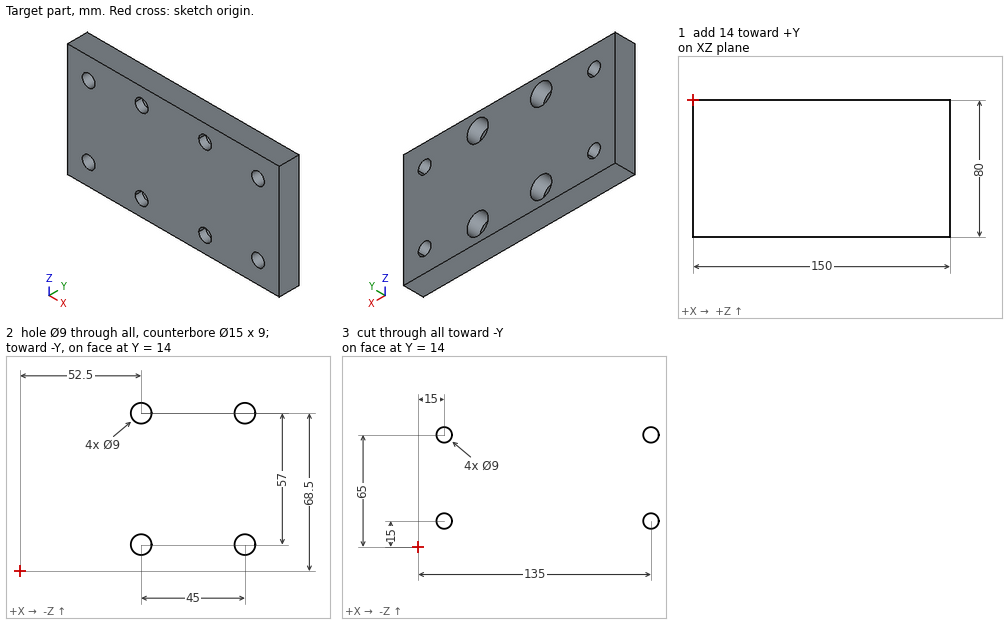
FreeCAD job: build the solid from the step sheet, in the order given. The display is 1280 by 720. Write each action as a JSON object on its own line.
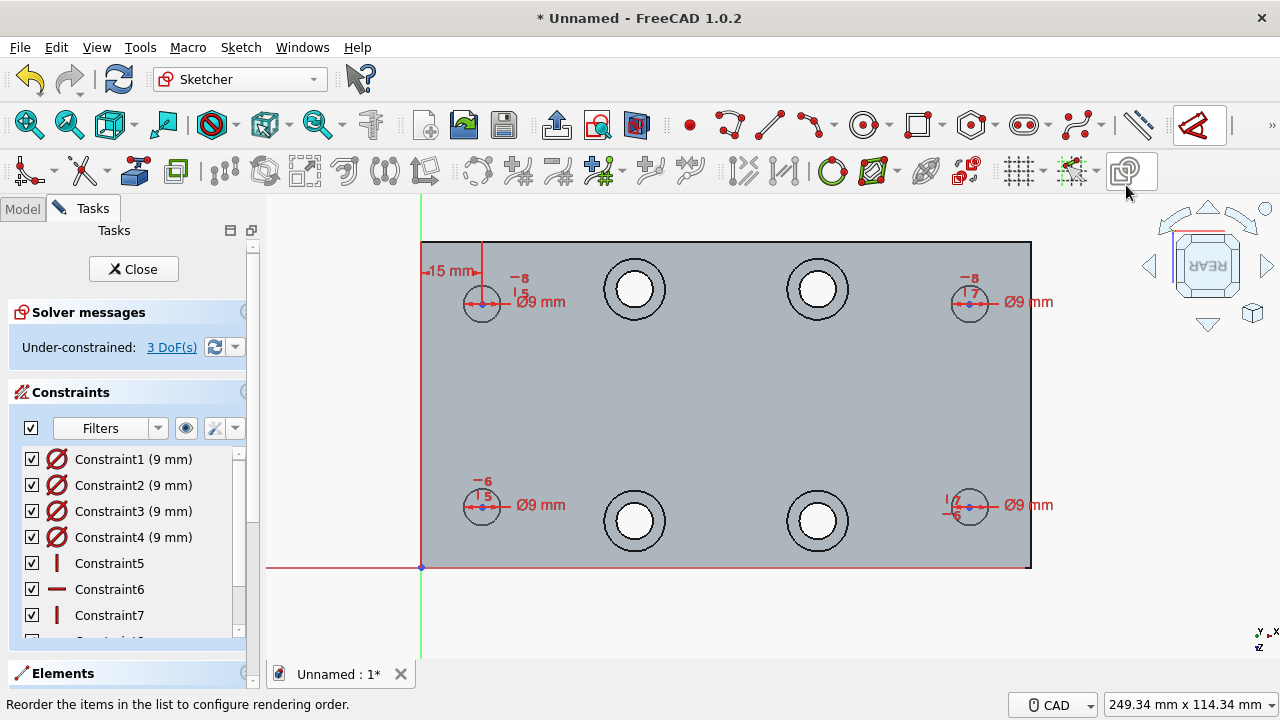
{"action": "left_click", "coordinate": [482, 304]}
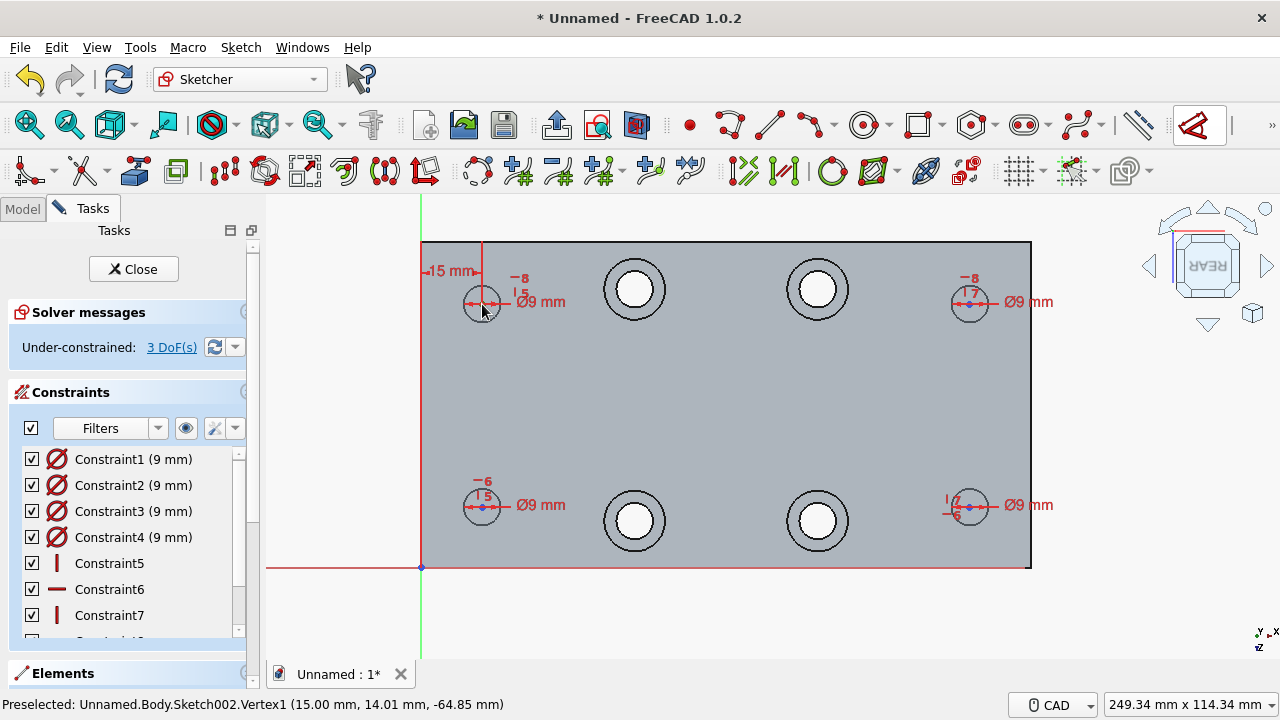
{"action": "left_click", "coordinate": [1220, 126]}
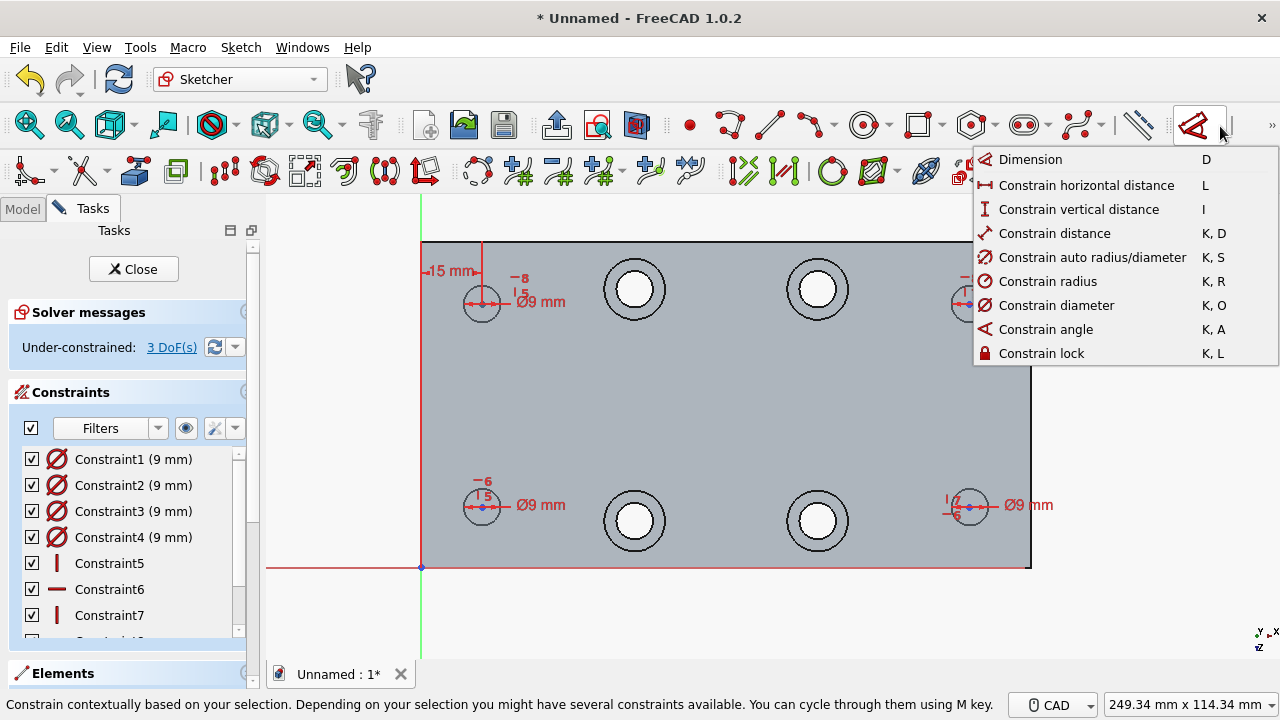
{"action": "left_click", "coordinate": [1126, 209]}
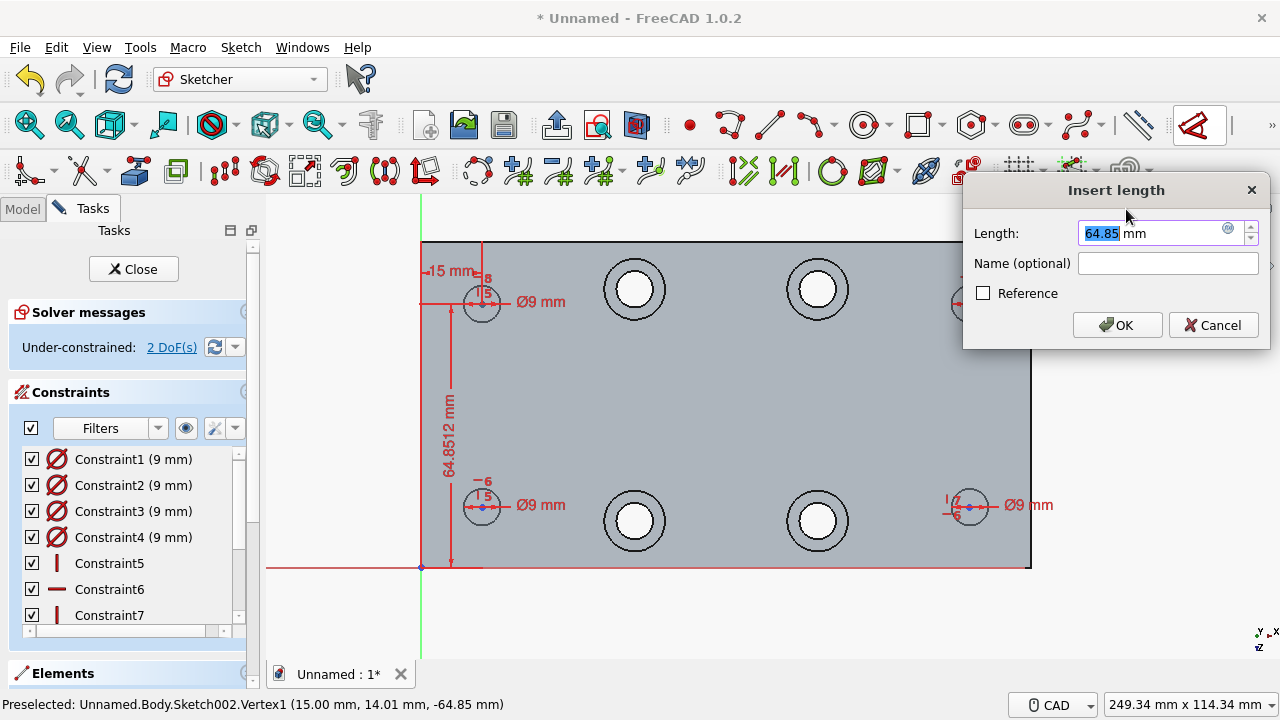
{"action": "type", "text": "65"}
{"action": "key", "text": "Return"}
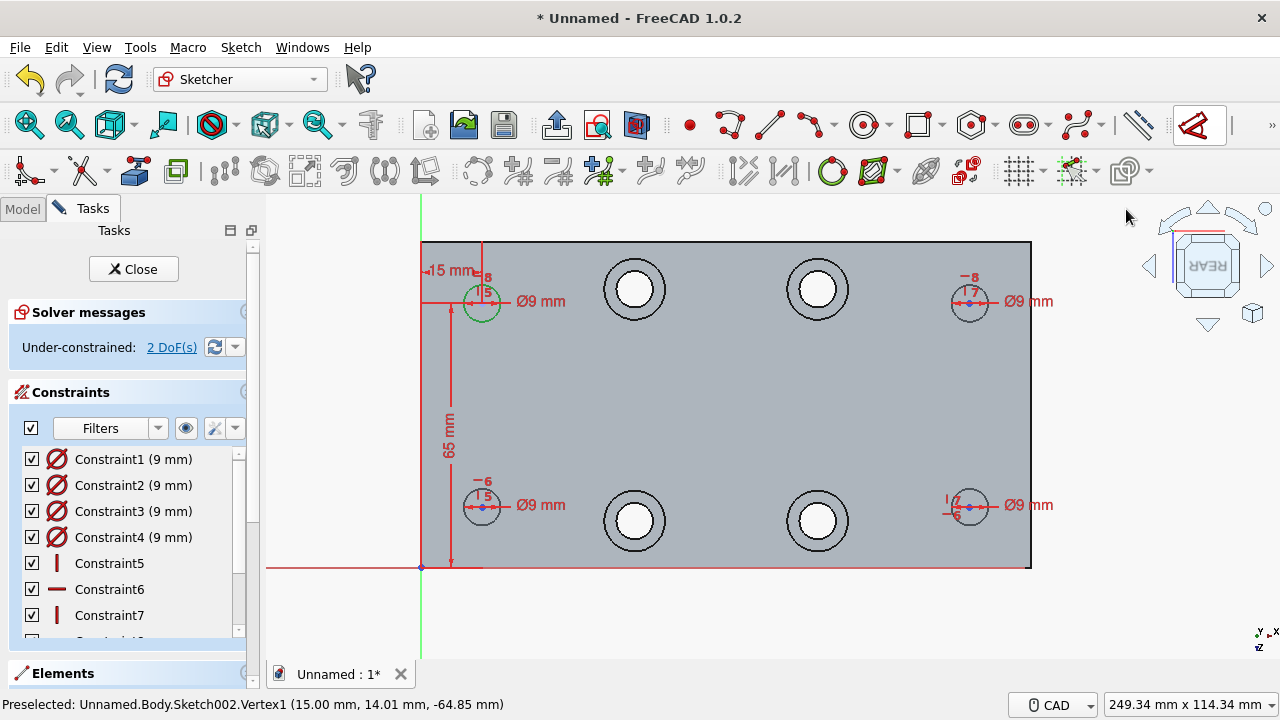
{"action": "left_click", "coordinate": [482, 507]}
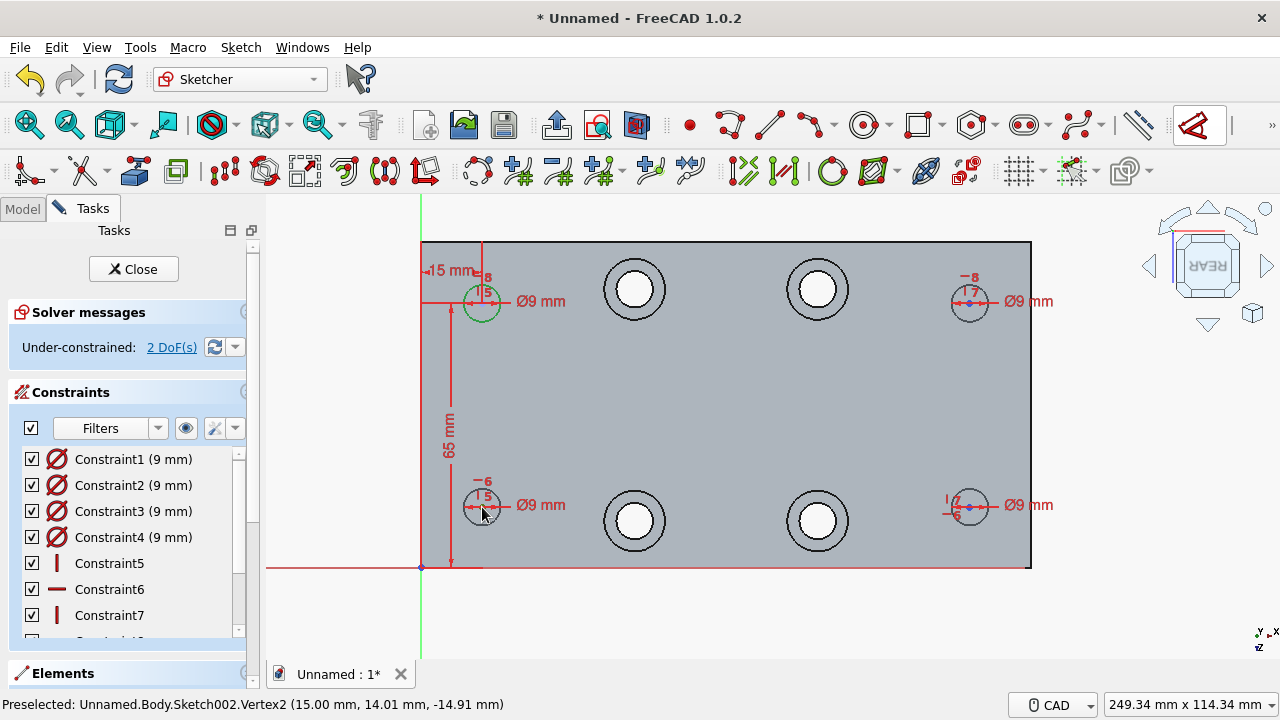
{"action": "key", "text": "i"}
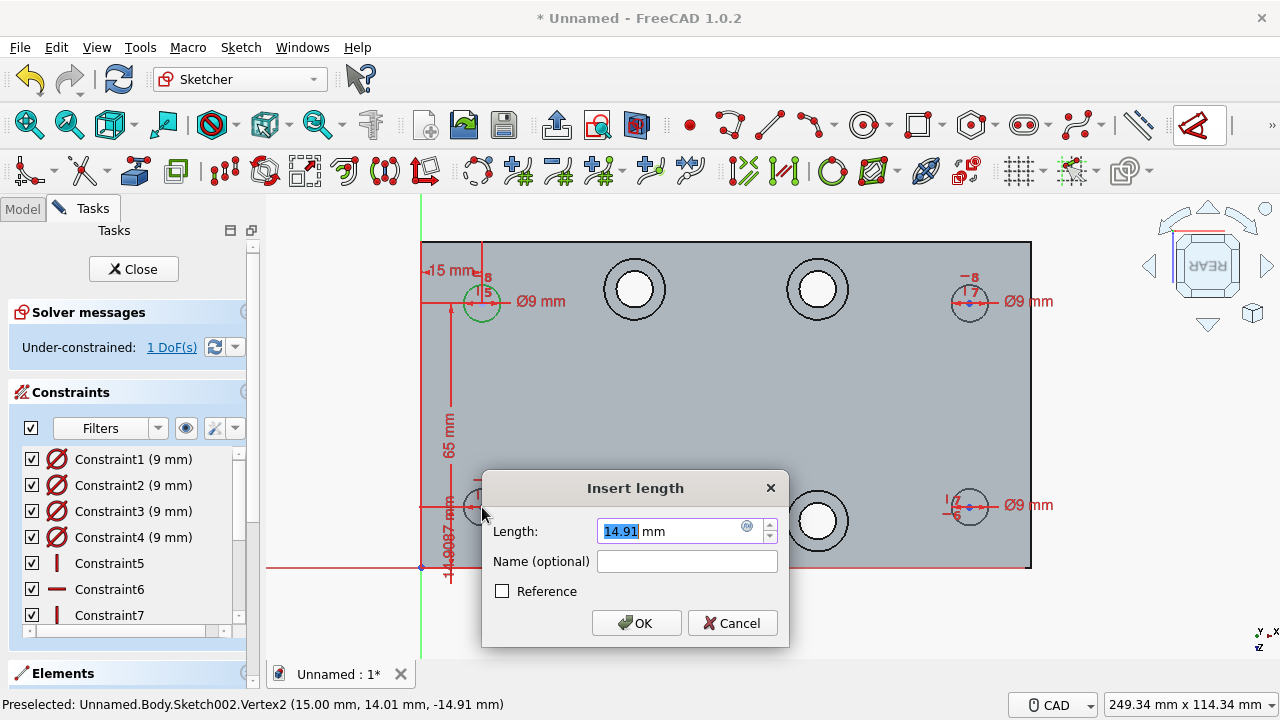
{"action": "type", "text": "15"}
{"action": "key", "text": "Return"}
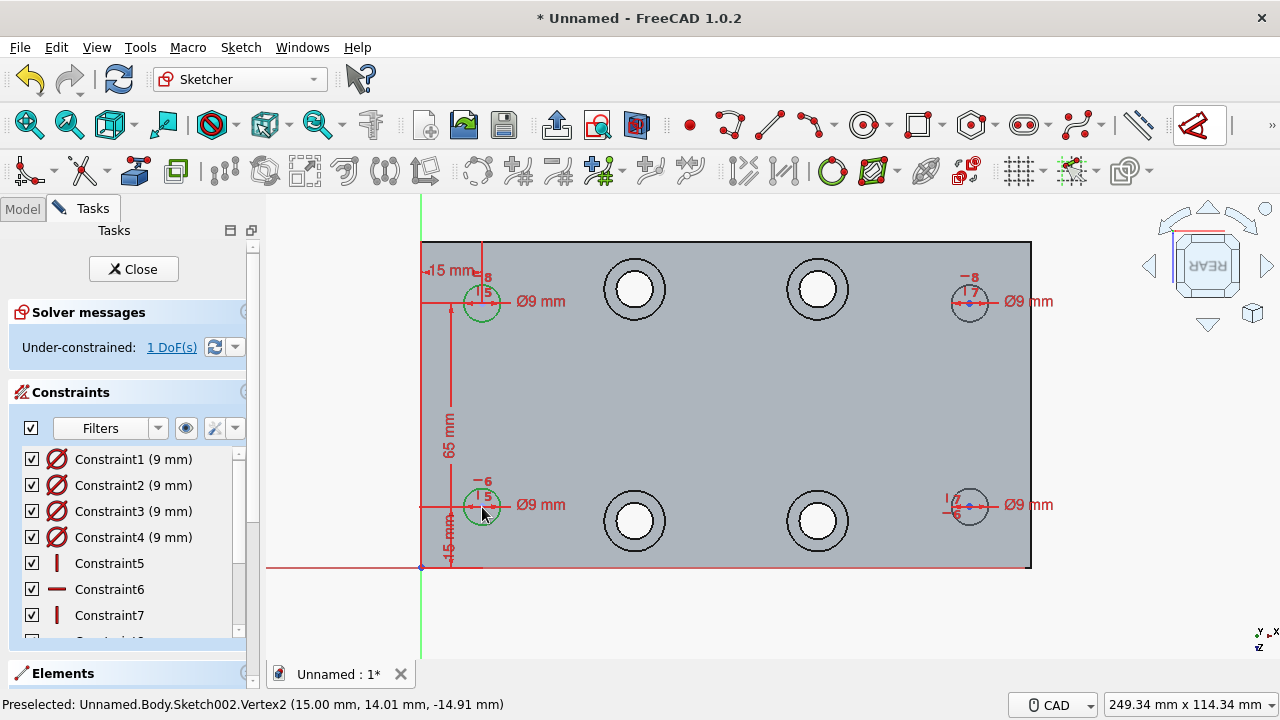
{"action": "left_click", "coordinate": [970, 507]}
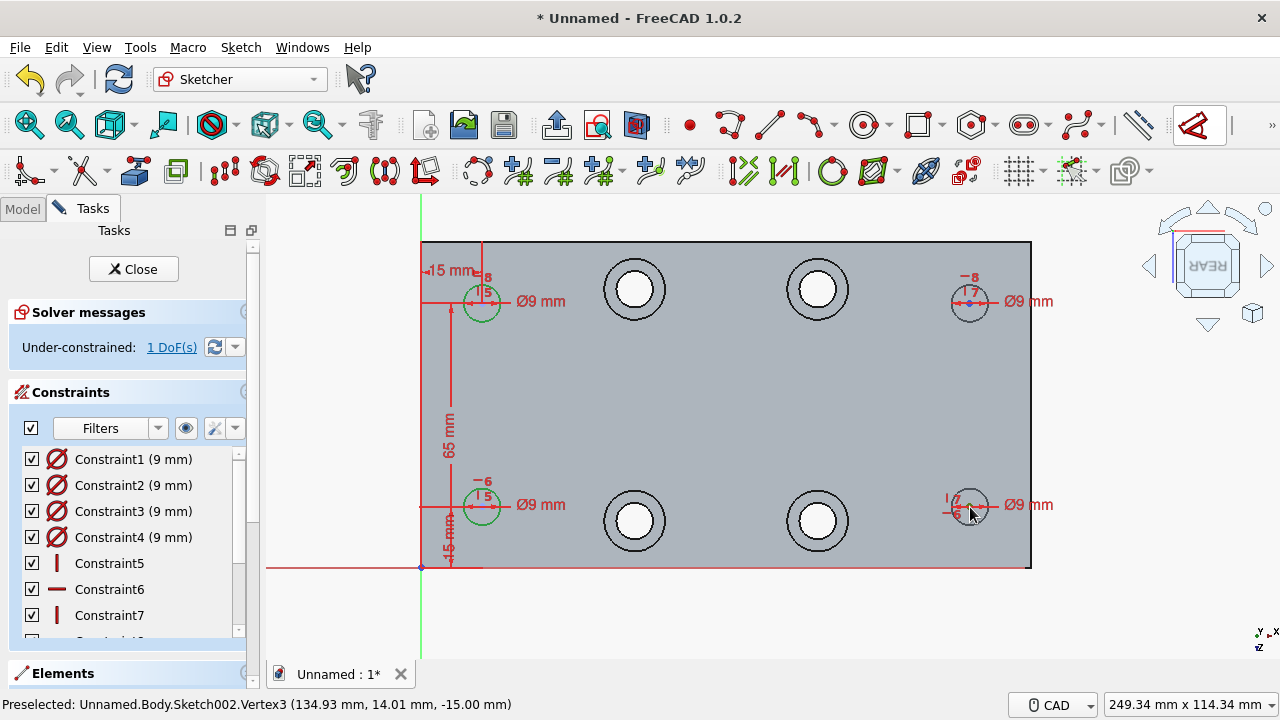
{"action": "left_click", "coordinate": [1220, 126]}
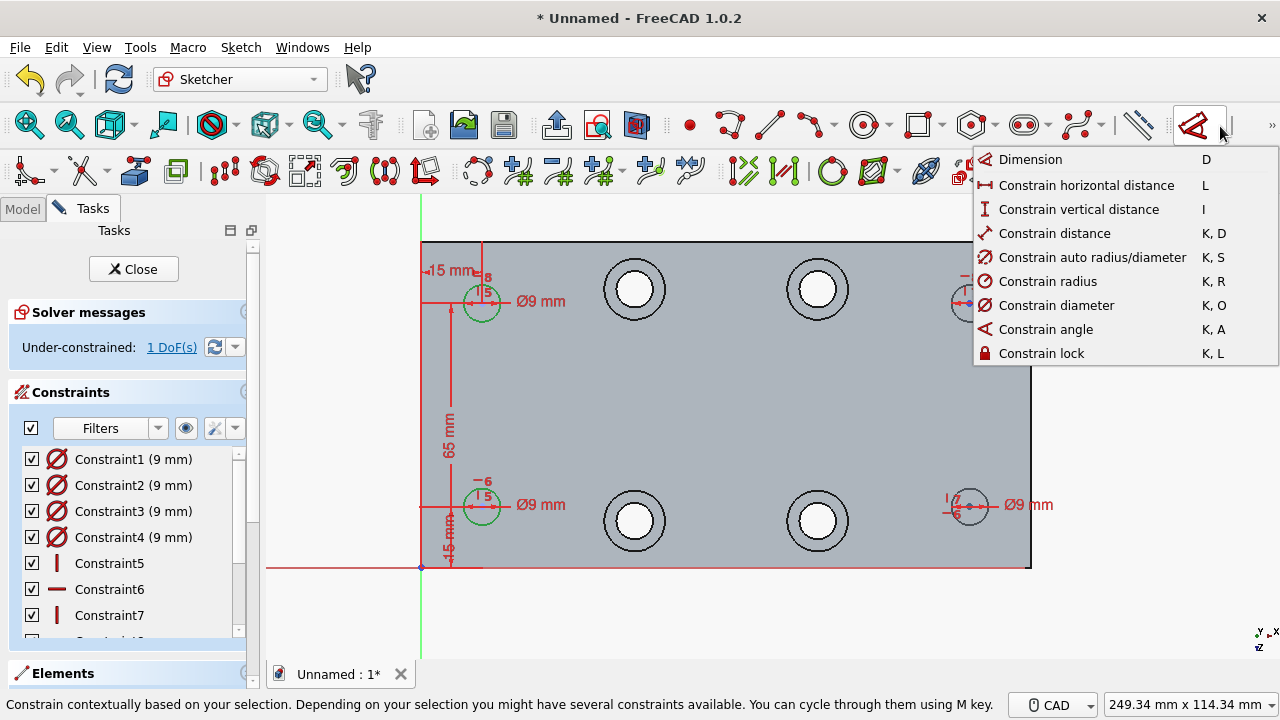
{"action": "left_click", "coordinate": [1126, 185]}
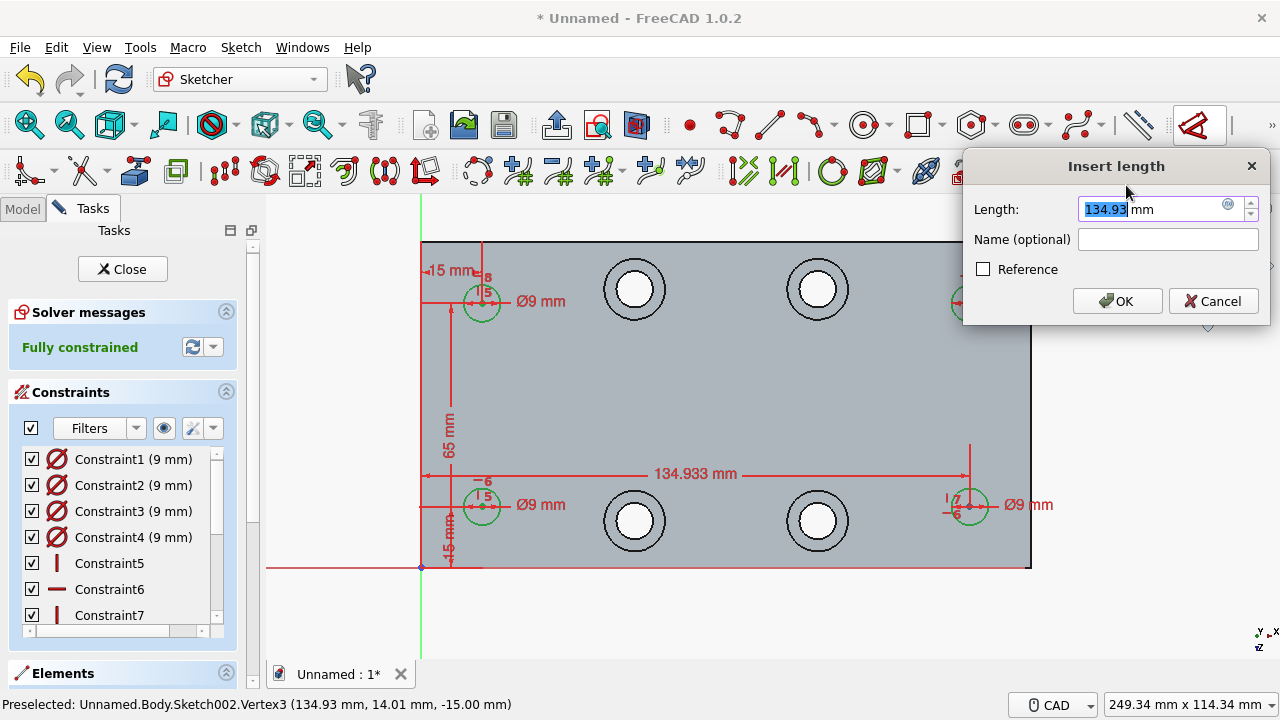
{"action": "type", "text": "135"}
{"action": "key", "text": "Return"}